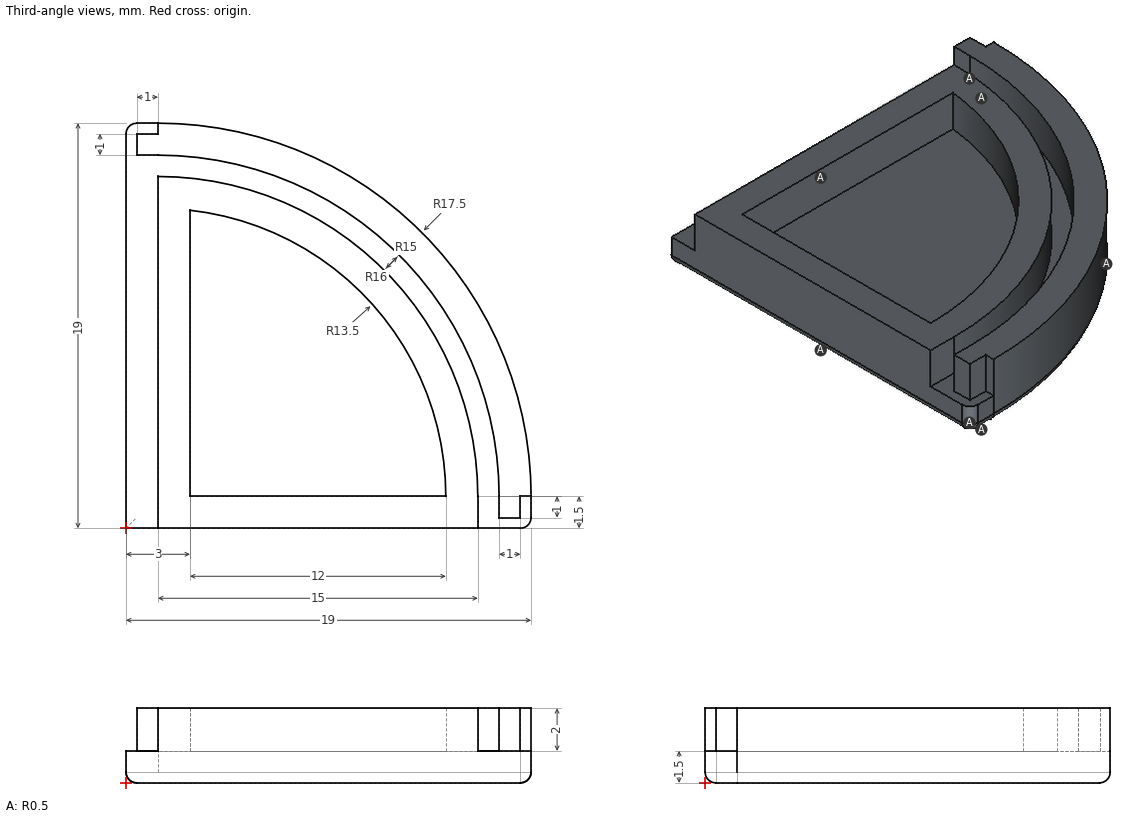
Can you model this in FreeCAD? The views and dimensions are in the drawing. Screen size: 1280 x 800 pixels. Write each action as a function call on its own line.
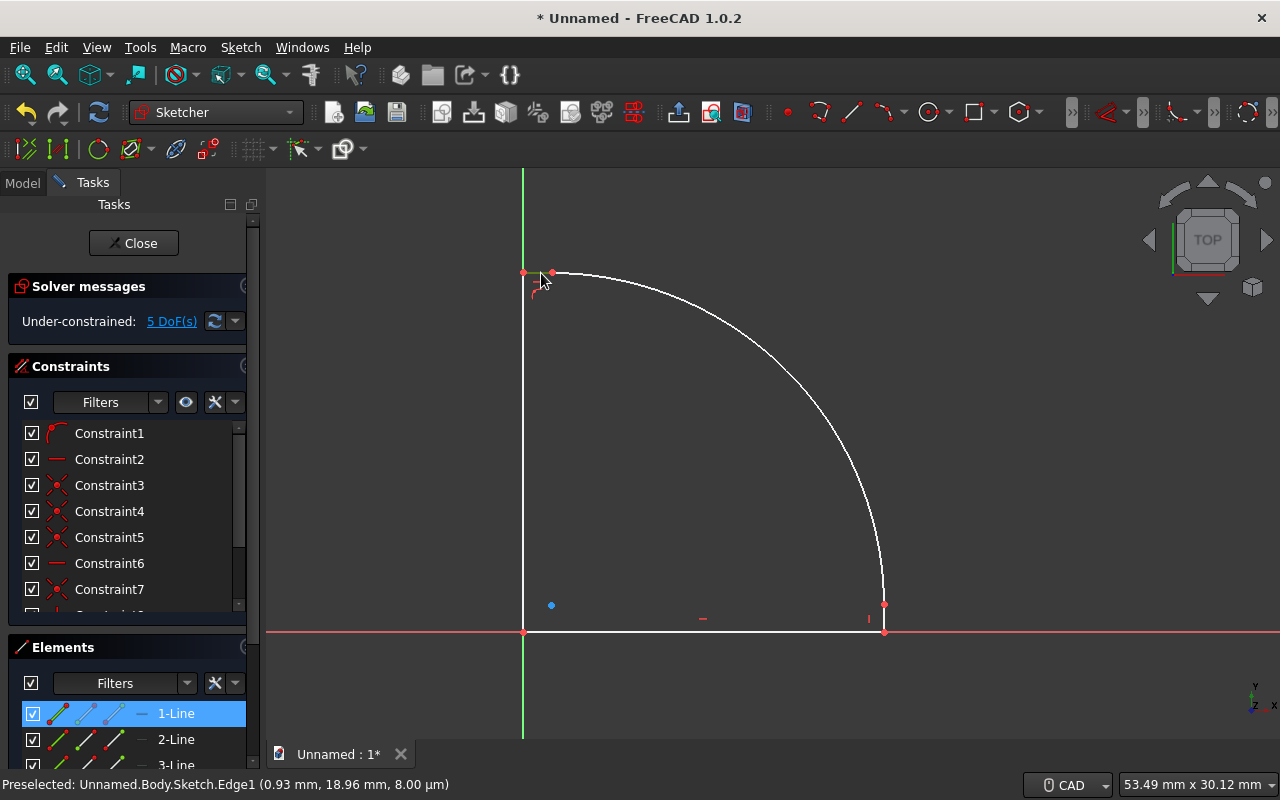
click(848, 454)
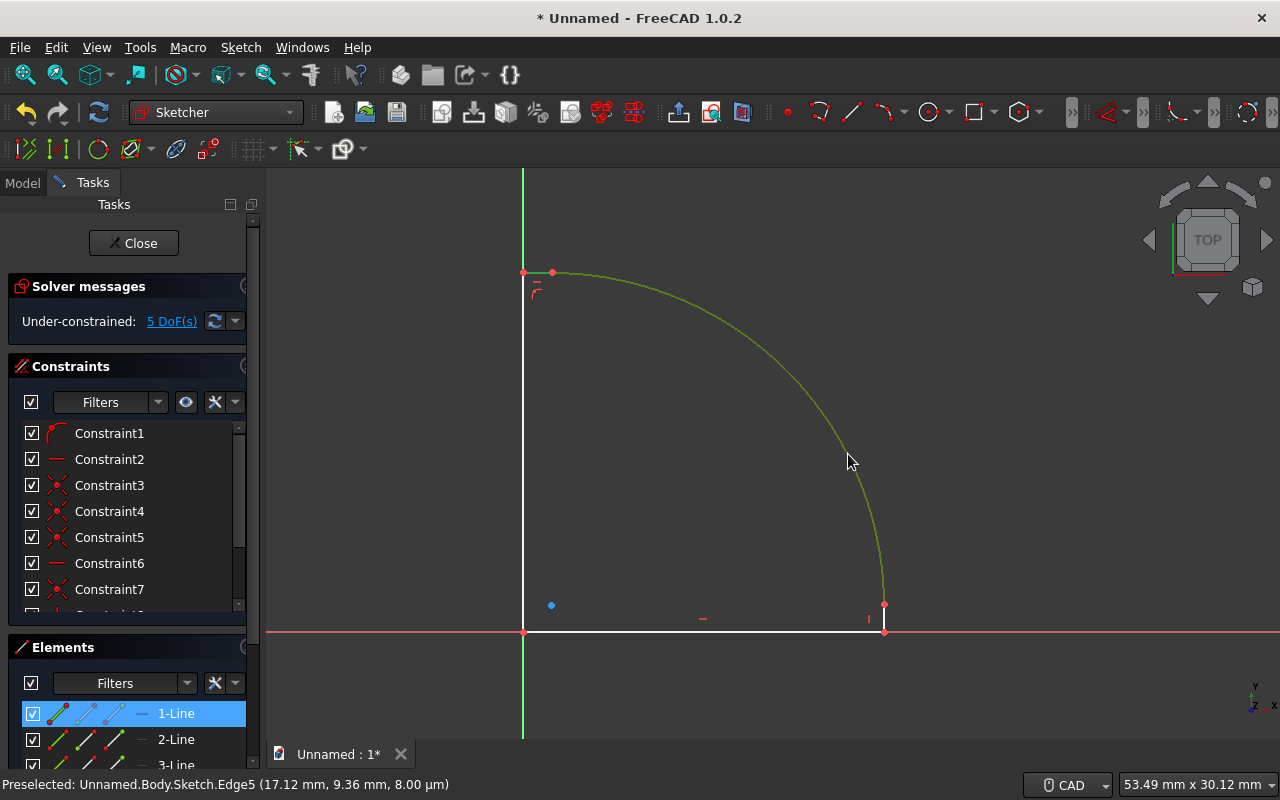
key(t)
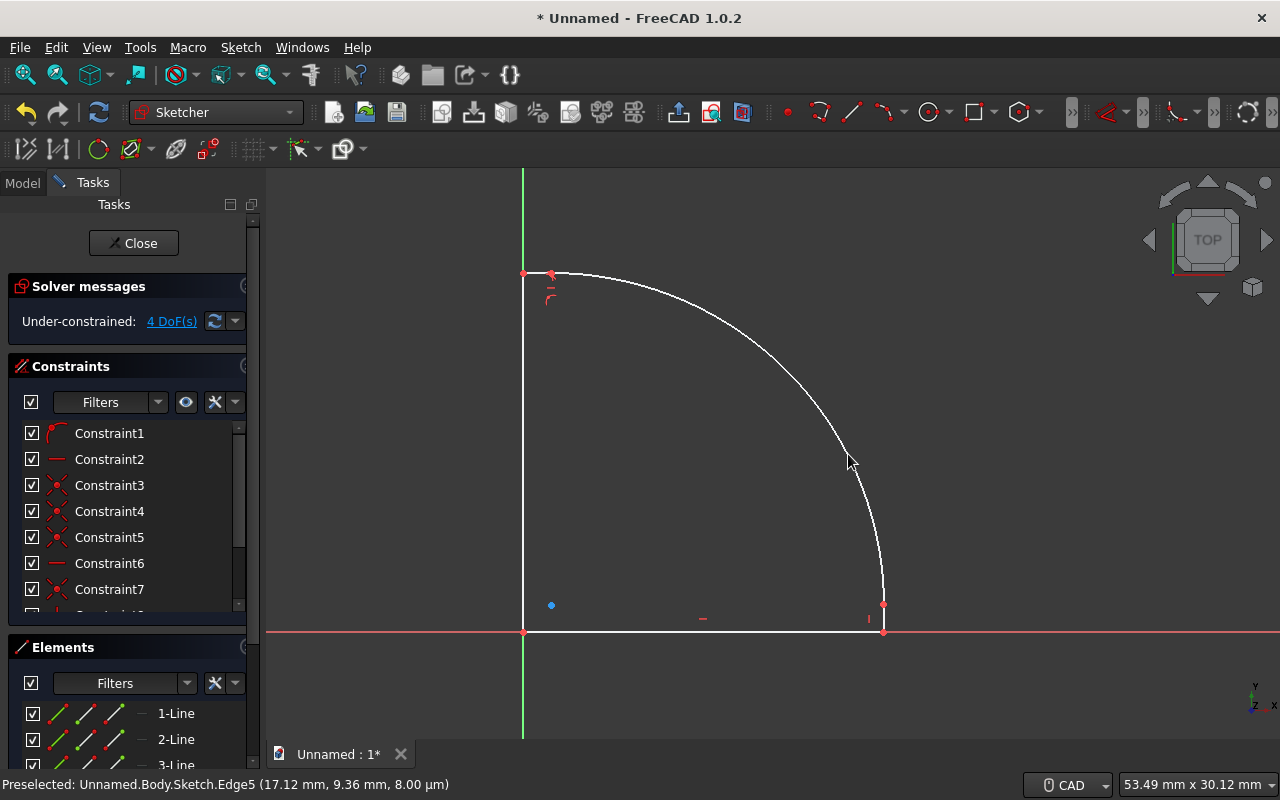
scroll(884, 621, up, 2)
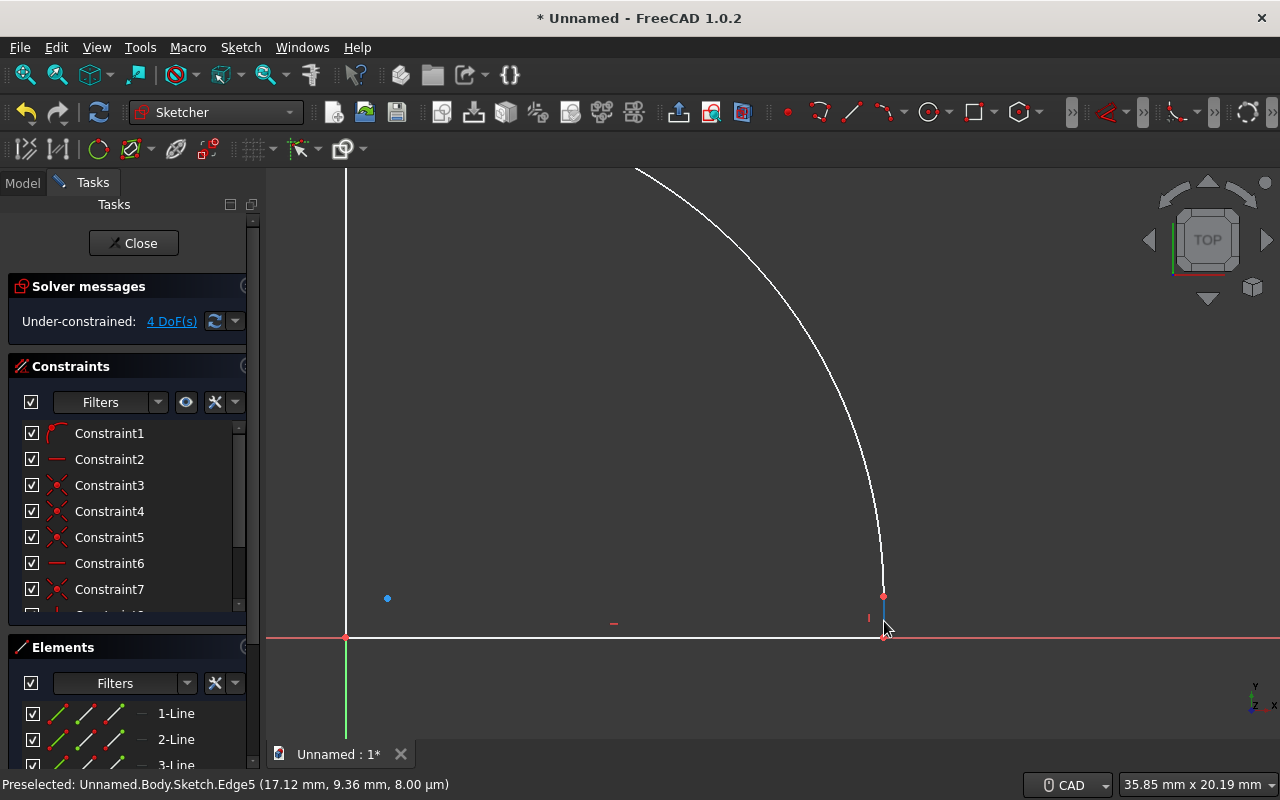
click(884, 621)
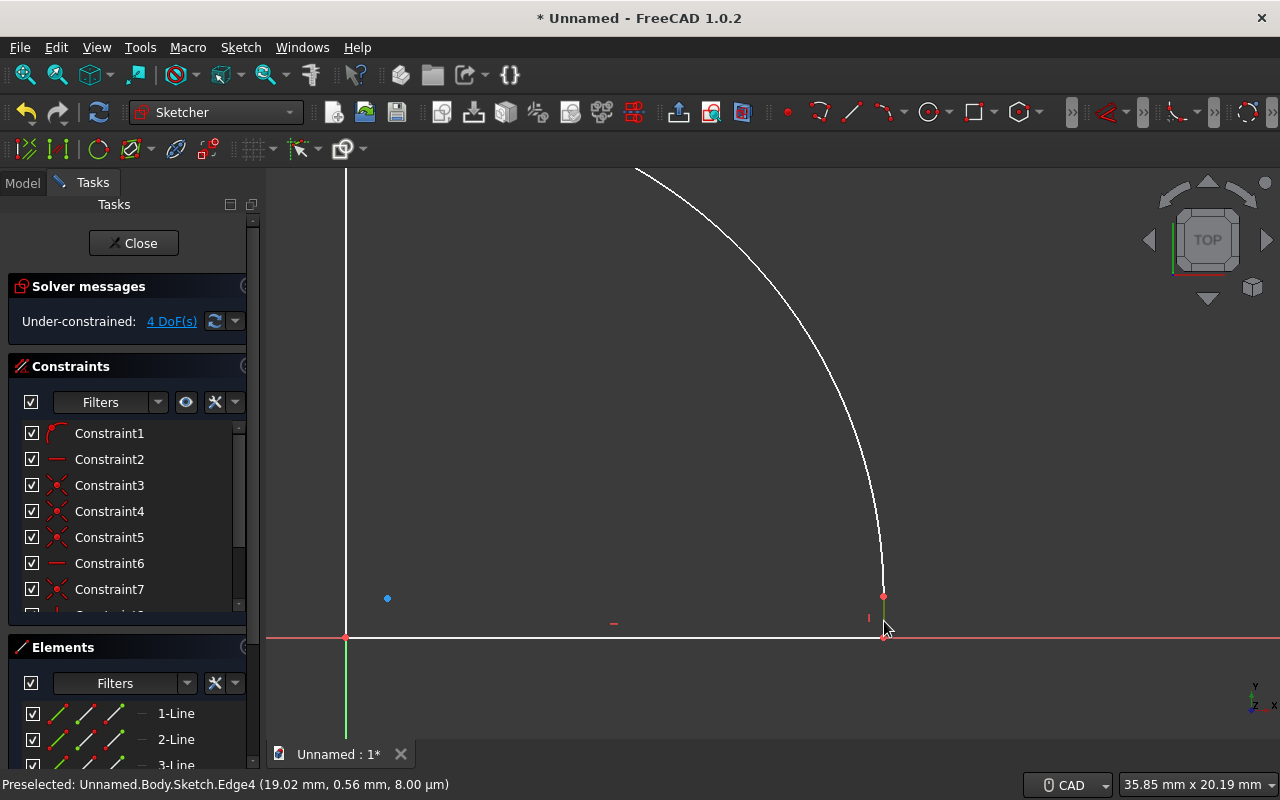
click(829, 372)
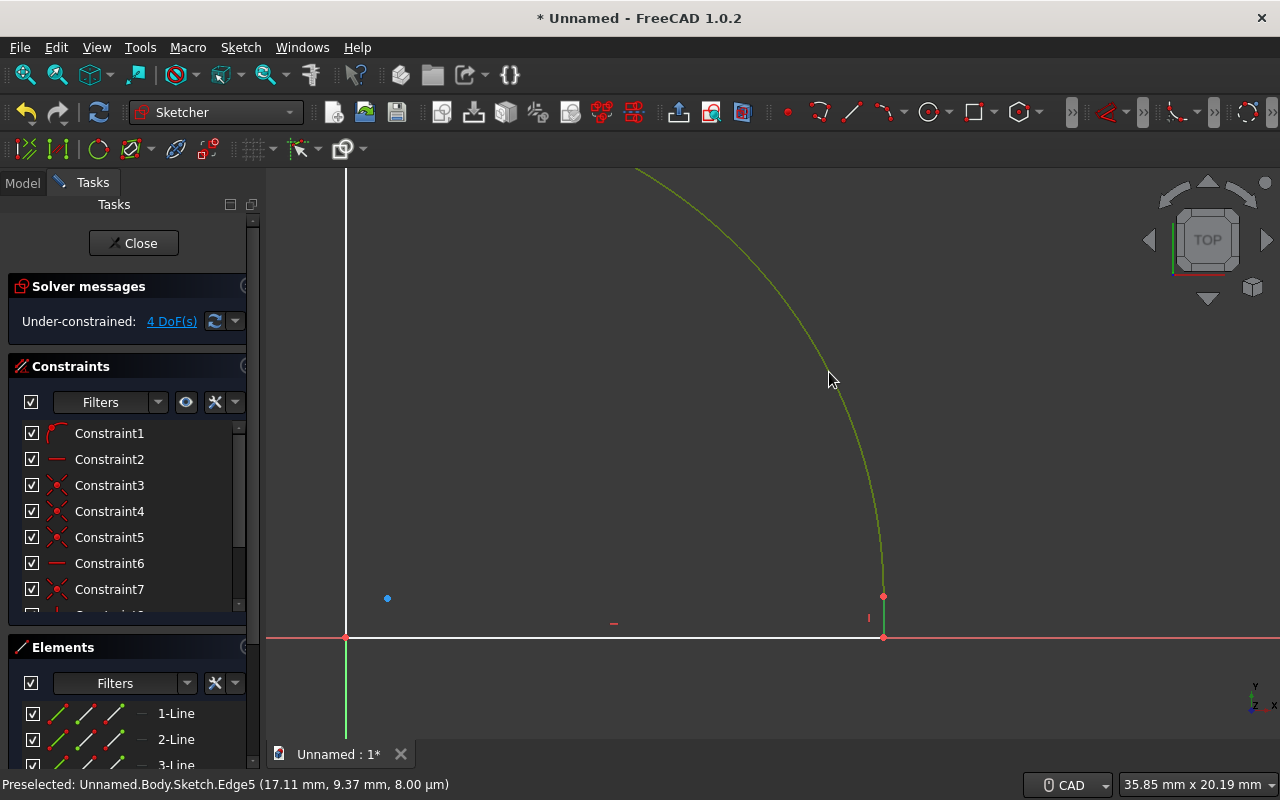
key(t)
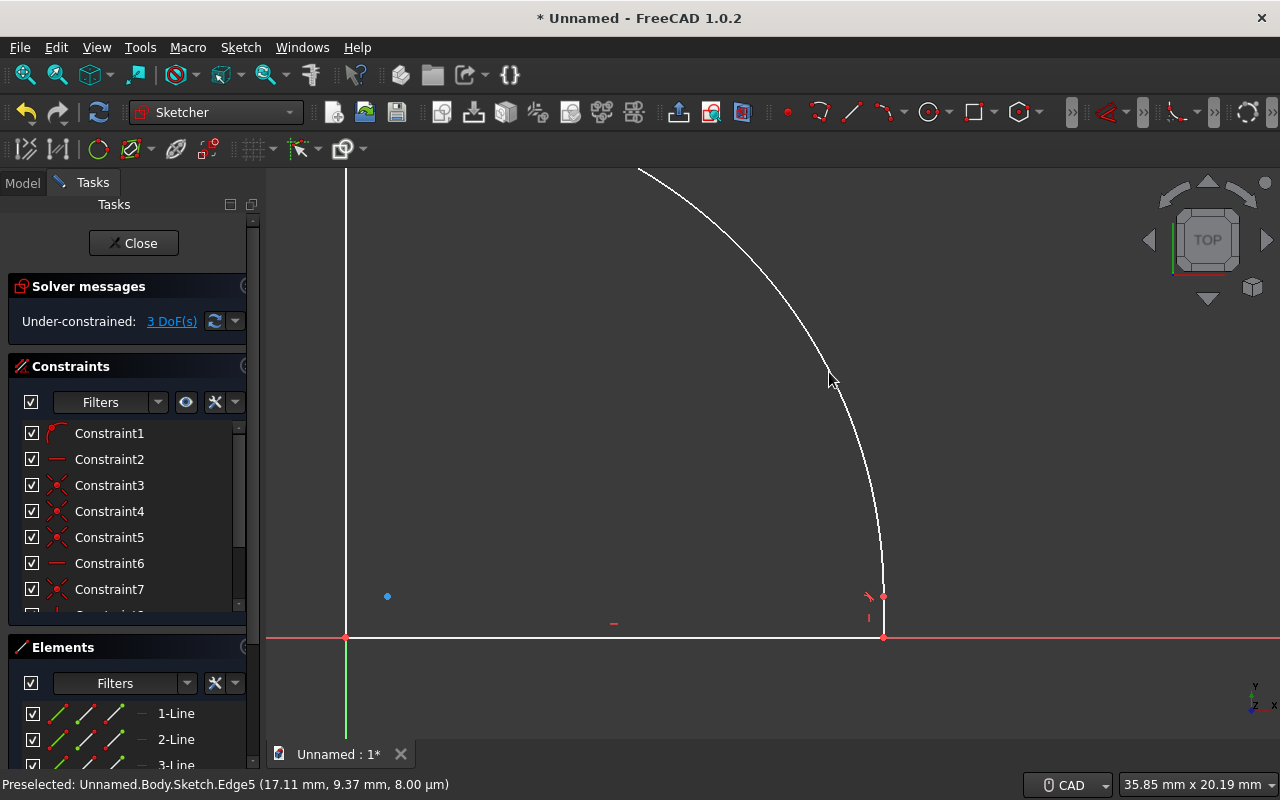
key(d)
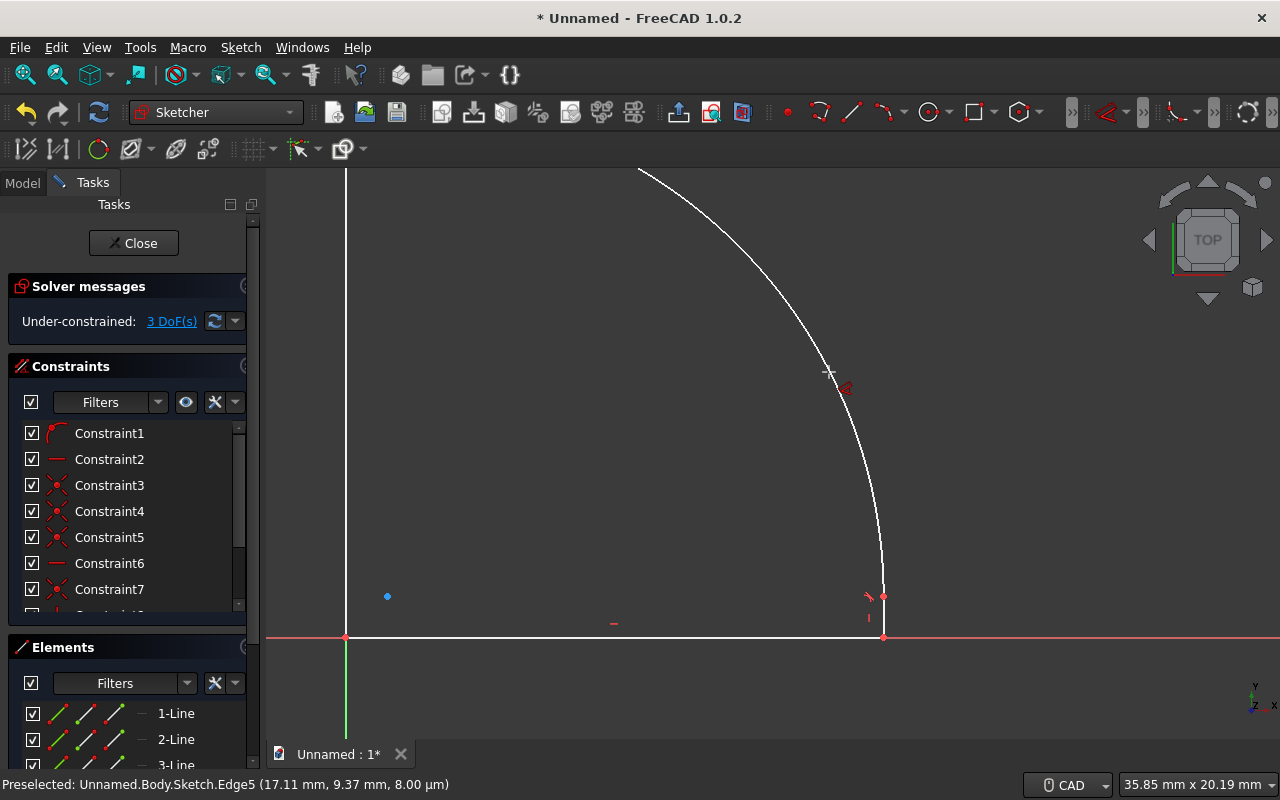
click(830, 371)
click(859, 356)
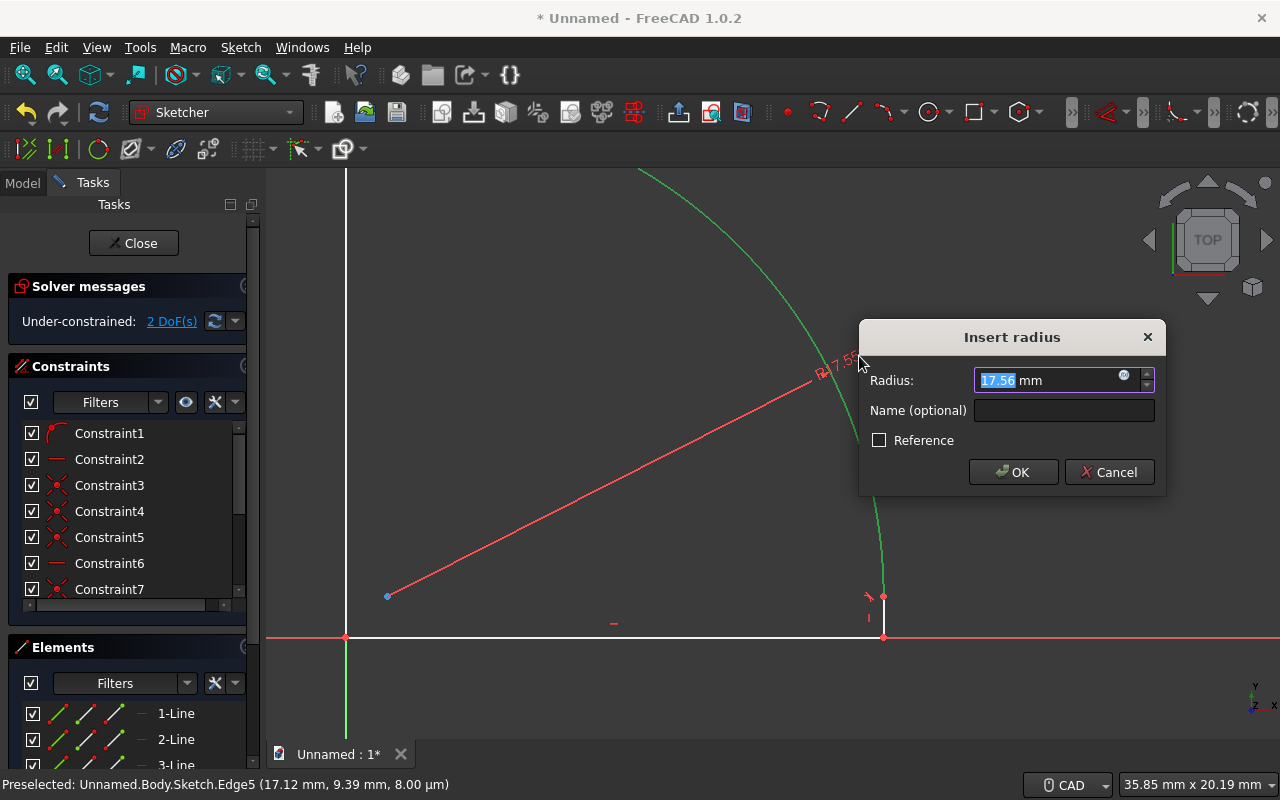
text(17.5)
key(Return)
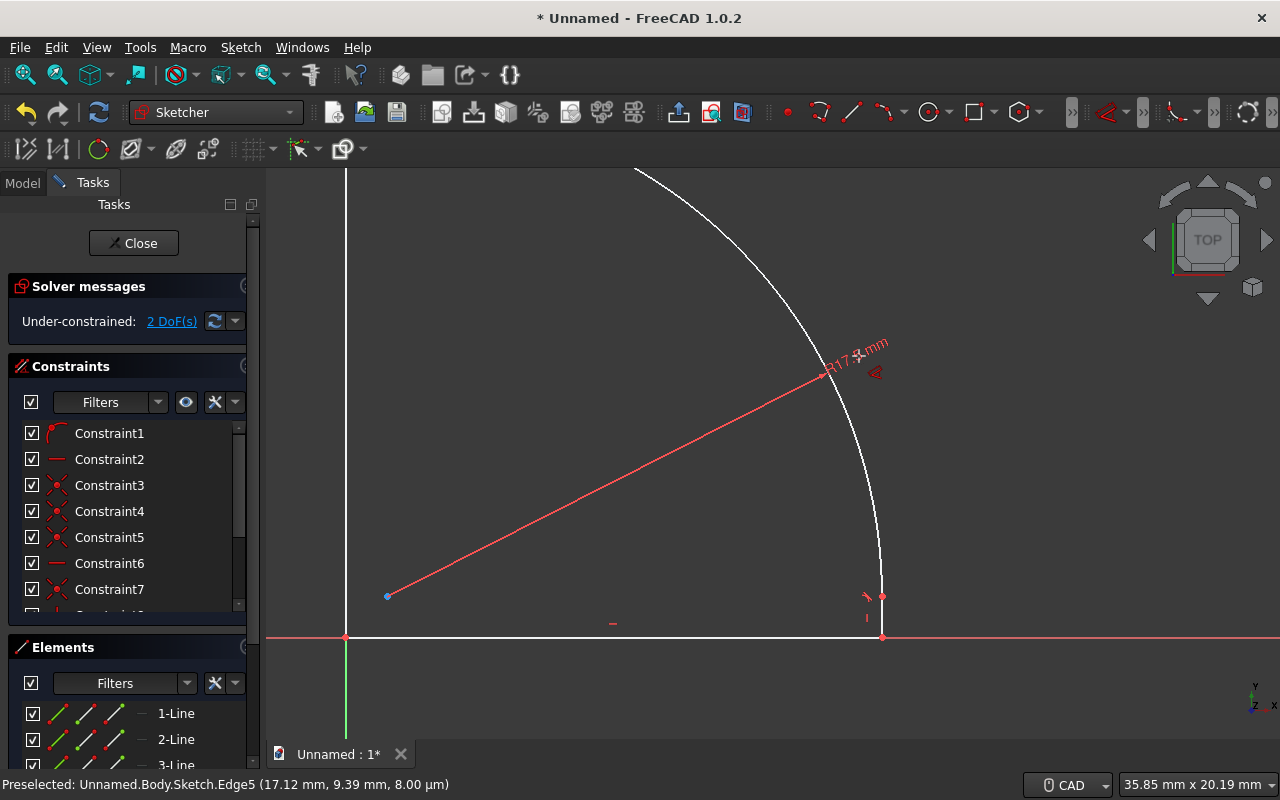
click(346, 263)
click(312, 417)